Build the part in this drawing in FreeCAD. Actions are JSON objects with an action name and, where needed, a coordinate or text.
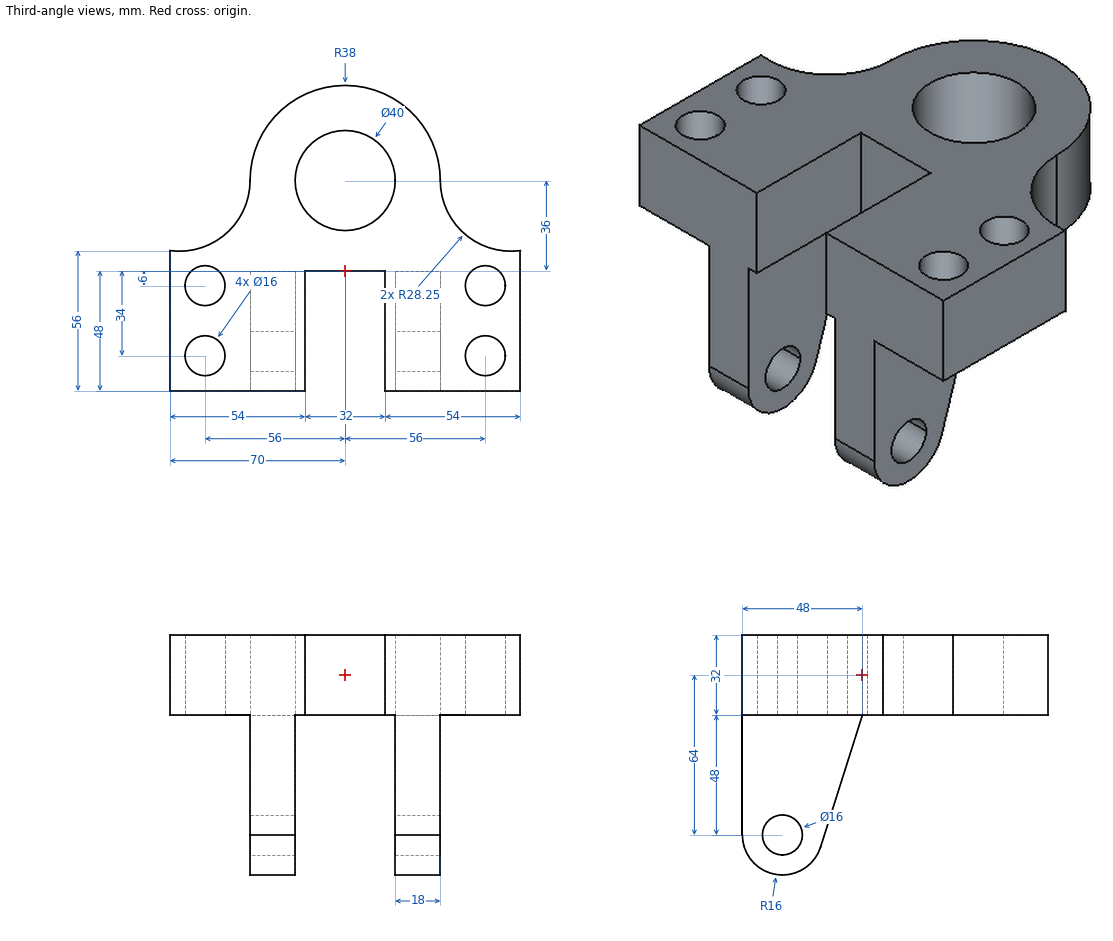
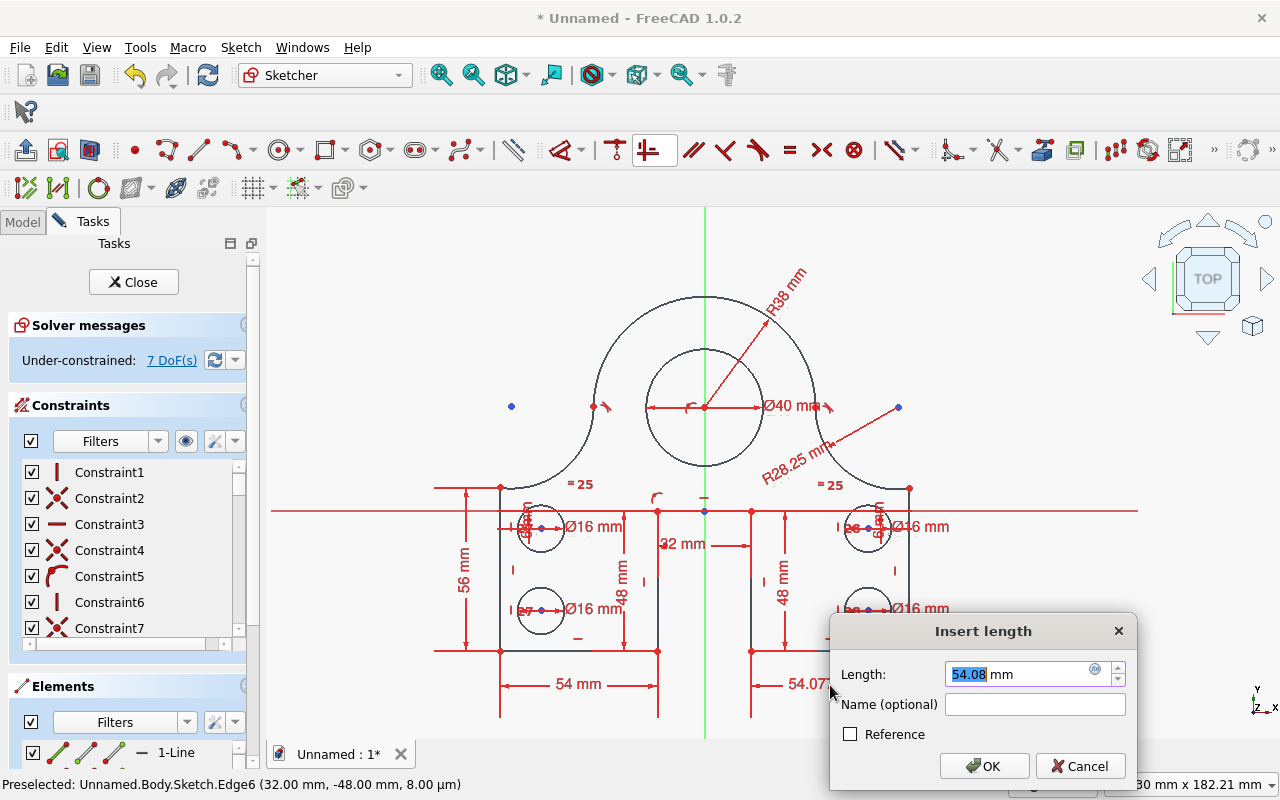
{"action": "type", "text": "54"}
{"action": "key", "text": "Return"}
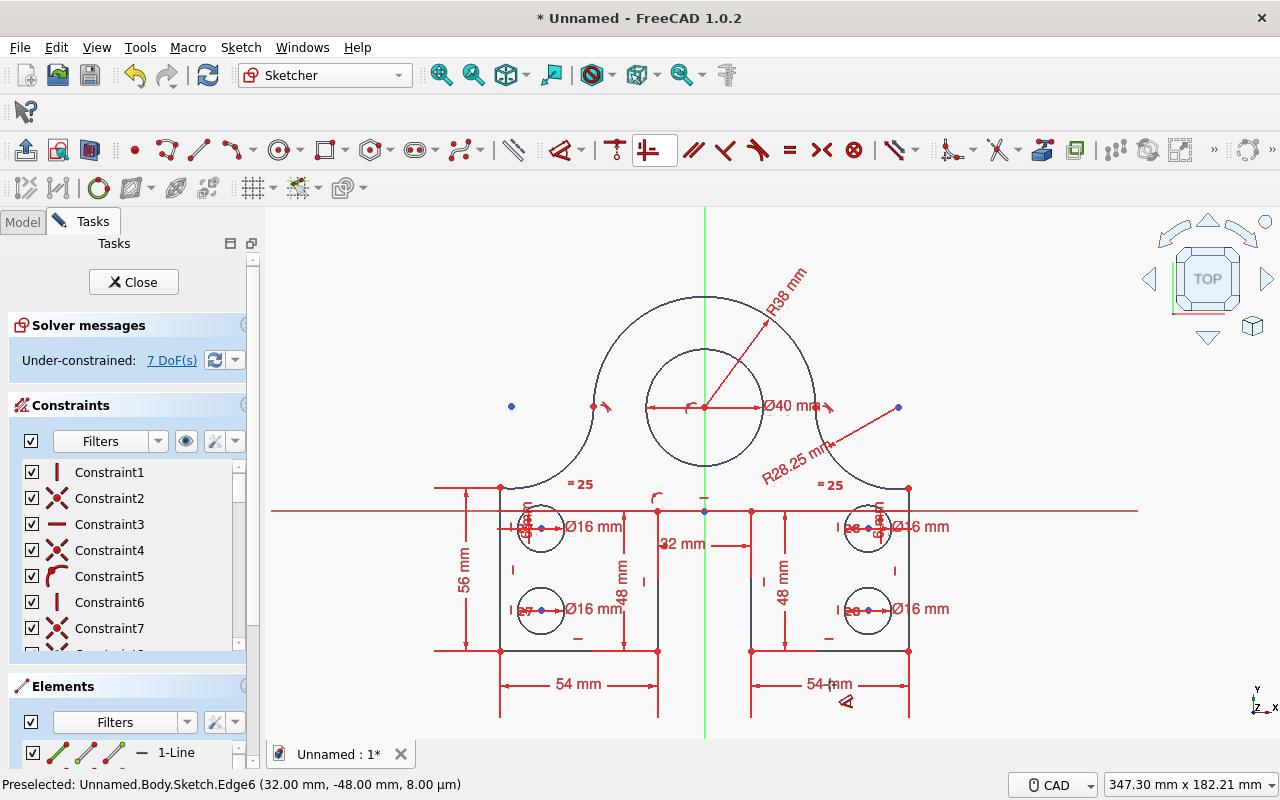
{"action": "left_click", "coordinate": [909, 603]}
{"action": "left_click", "coordinate": [943, 570]}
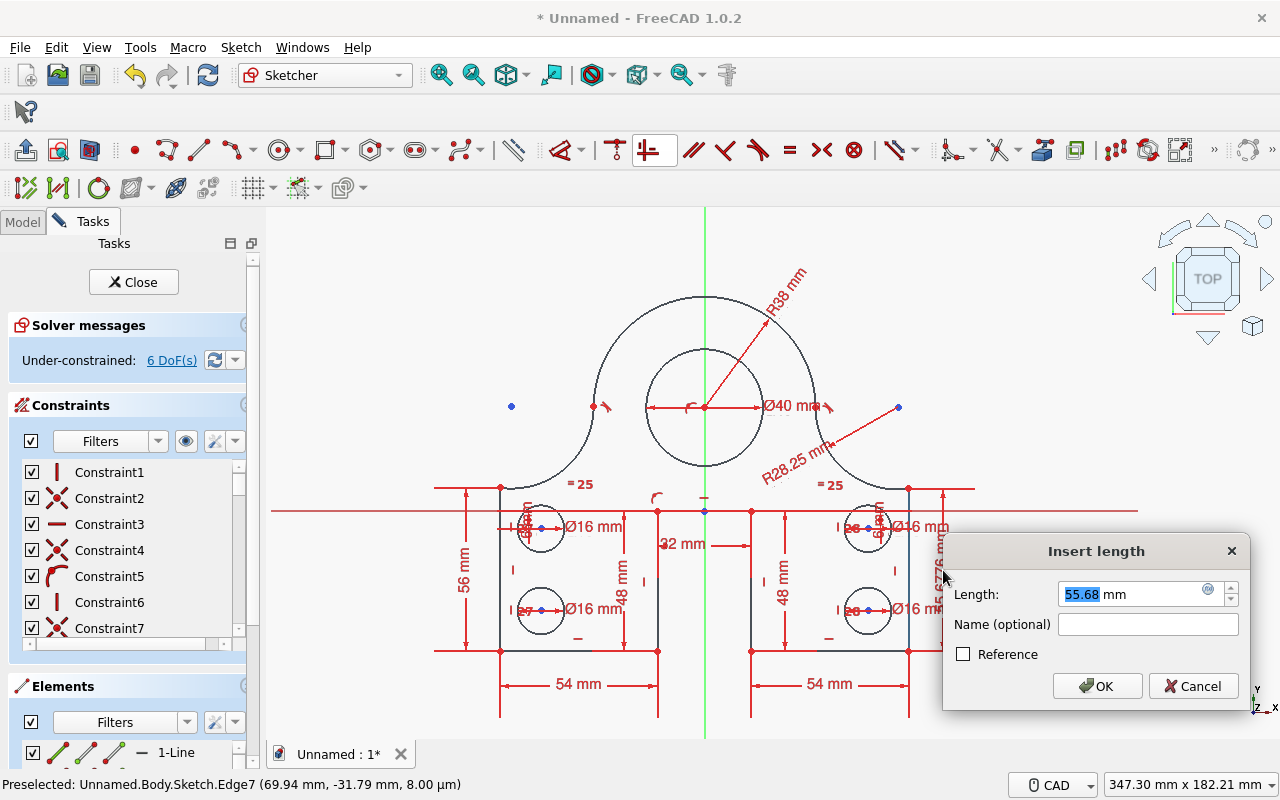
{"action": "type", "text": "56"}
{"action": "key", "text": "Return"}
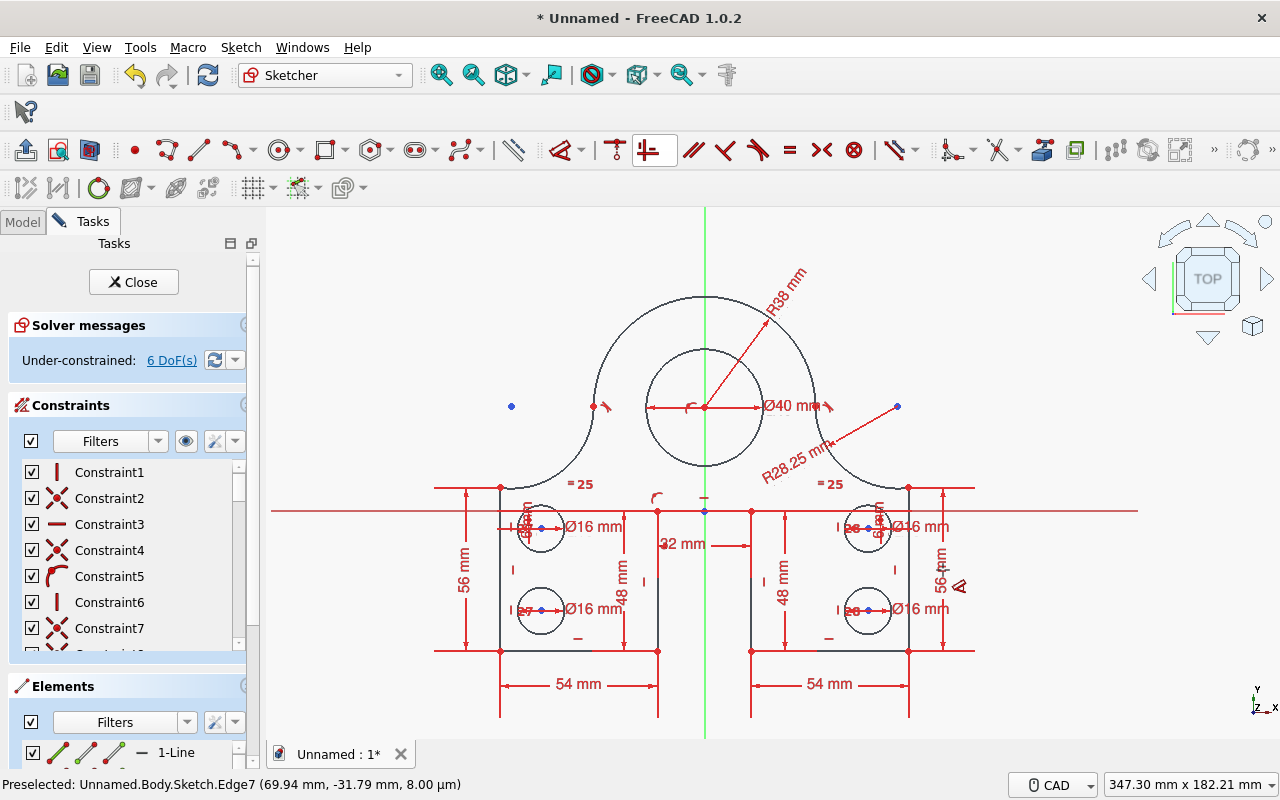
{"action": "left_click", "coordinate": [541, 611]}
{"action": "left_click", "coordinate": [680, 645]}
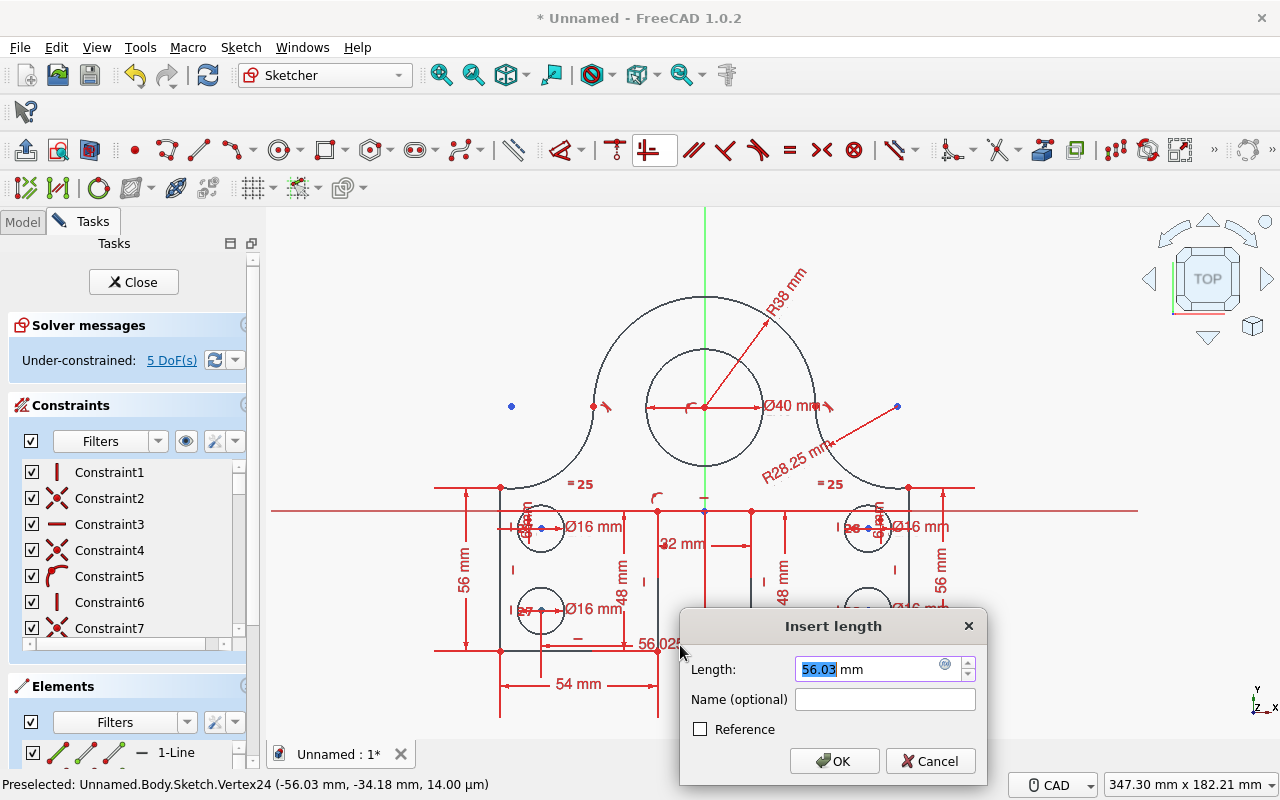
{"action": "type", "text": "56"}
{"action": "key", "text": "Return"}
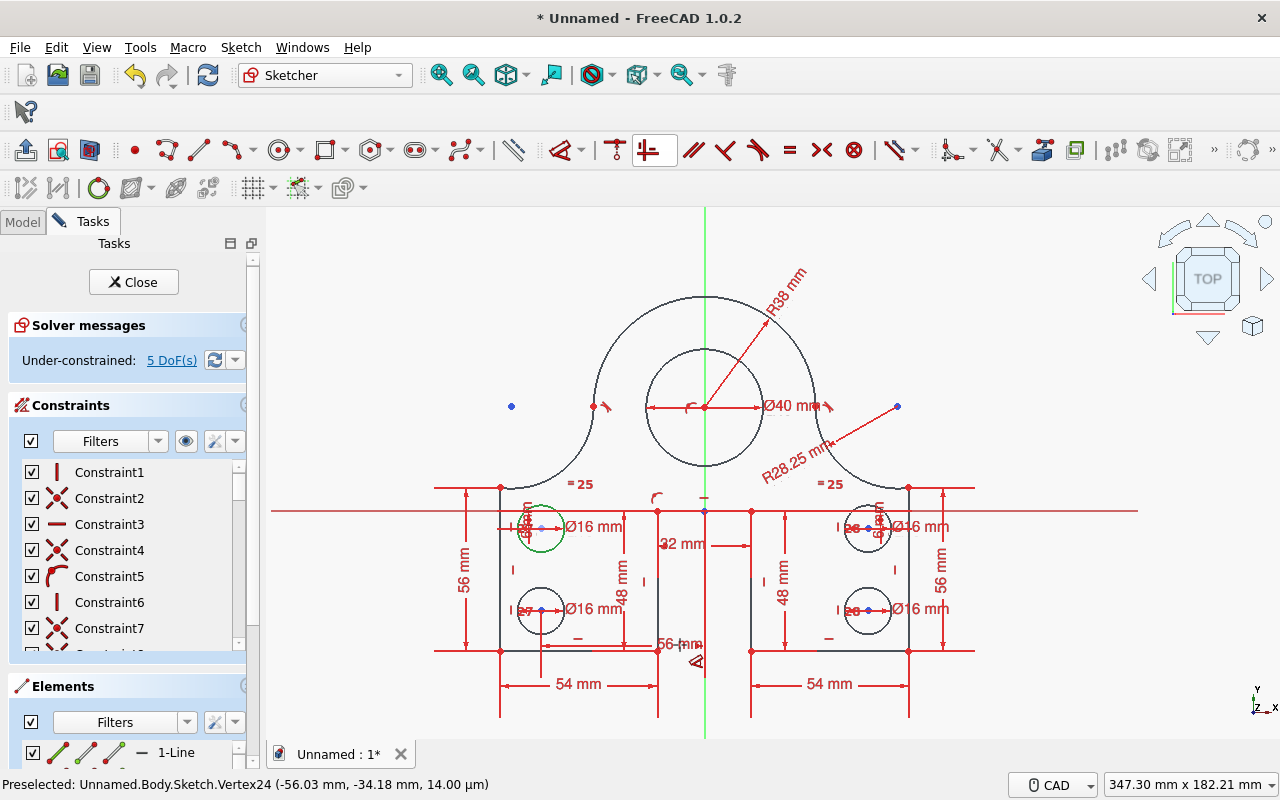
{"action": "left_click", "coordinate": [541, 611]}
{"action": "left_click", "coordinate": [483, 596]}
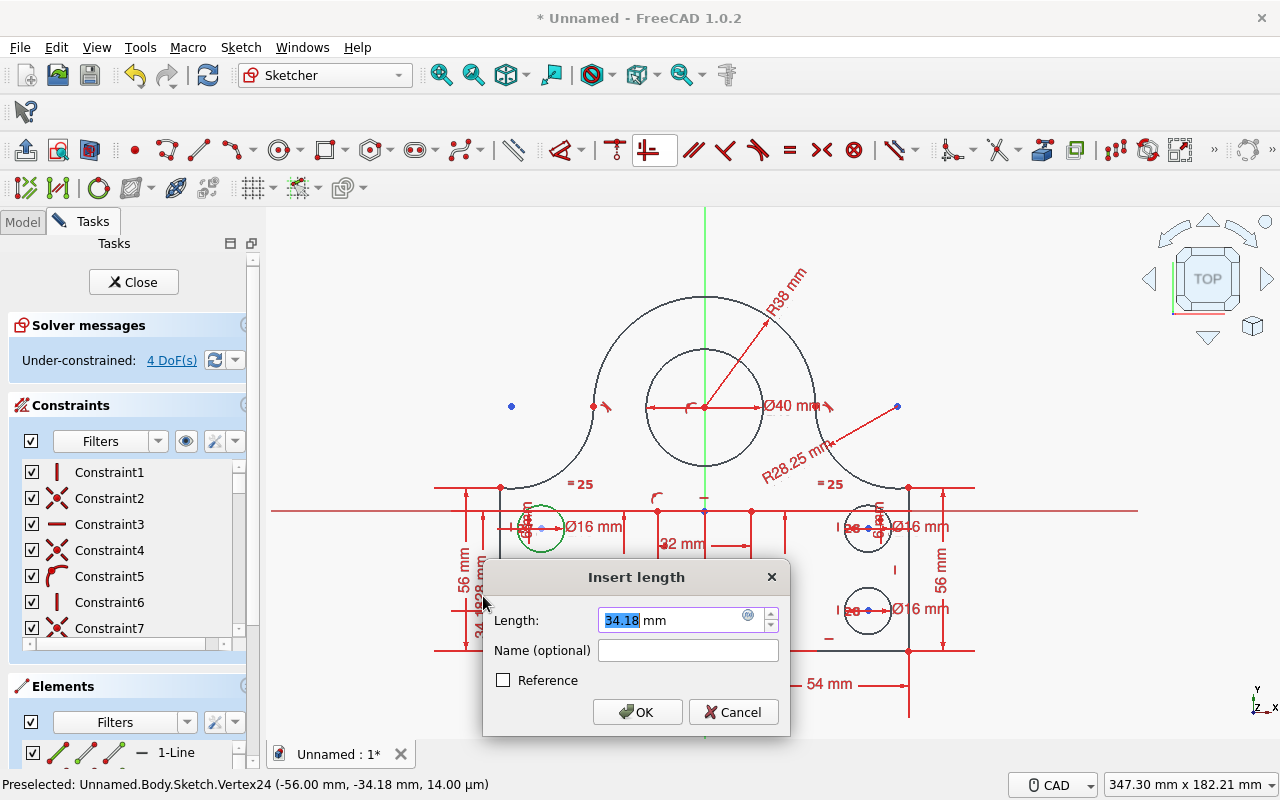
{"action": "type", "text": "34"}
{"action": "key", "text": "Return"}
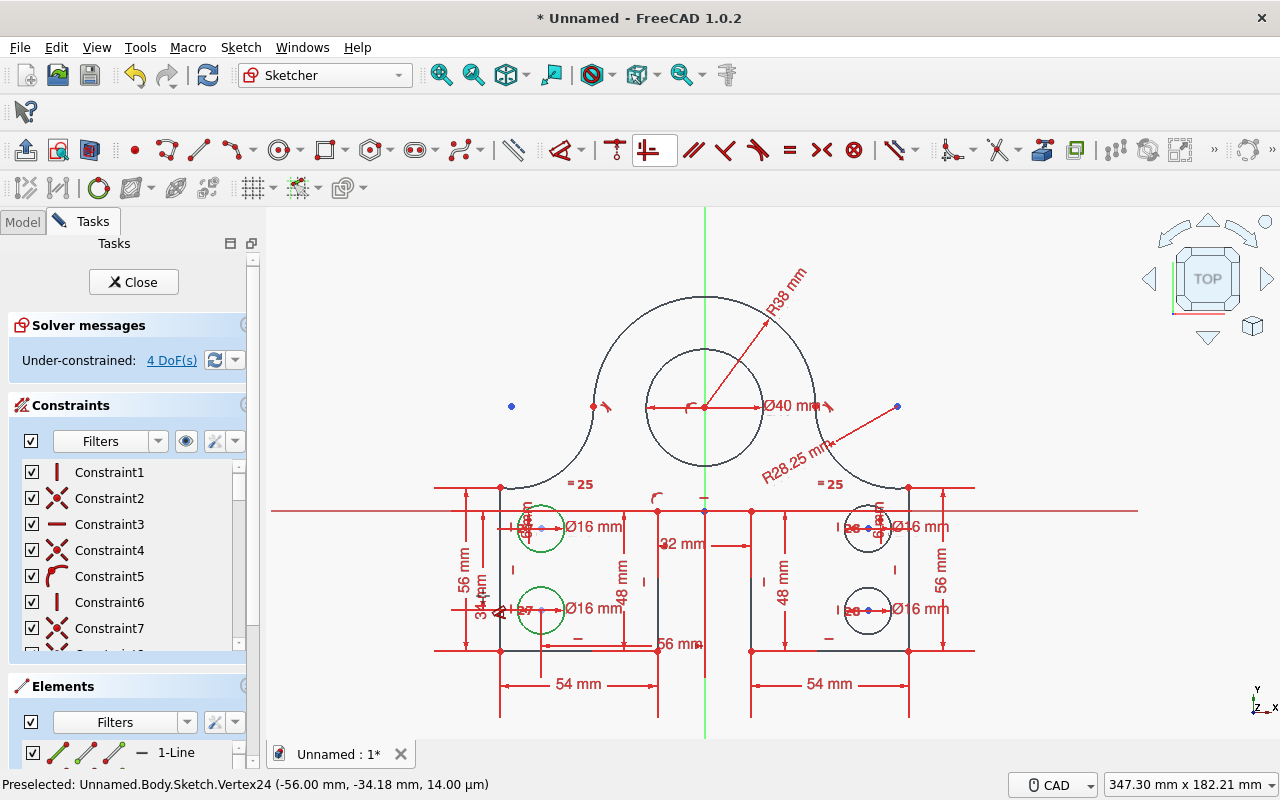
{"action": "left_click", "coordinate": [868, 611]}
{"action": "left_click", "coordinate": [749, 669]}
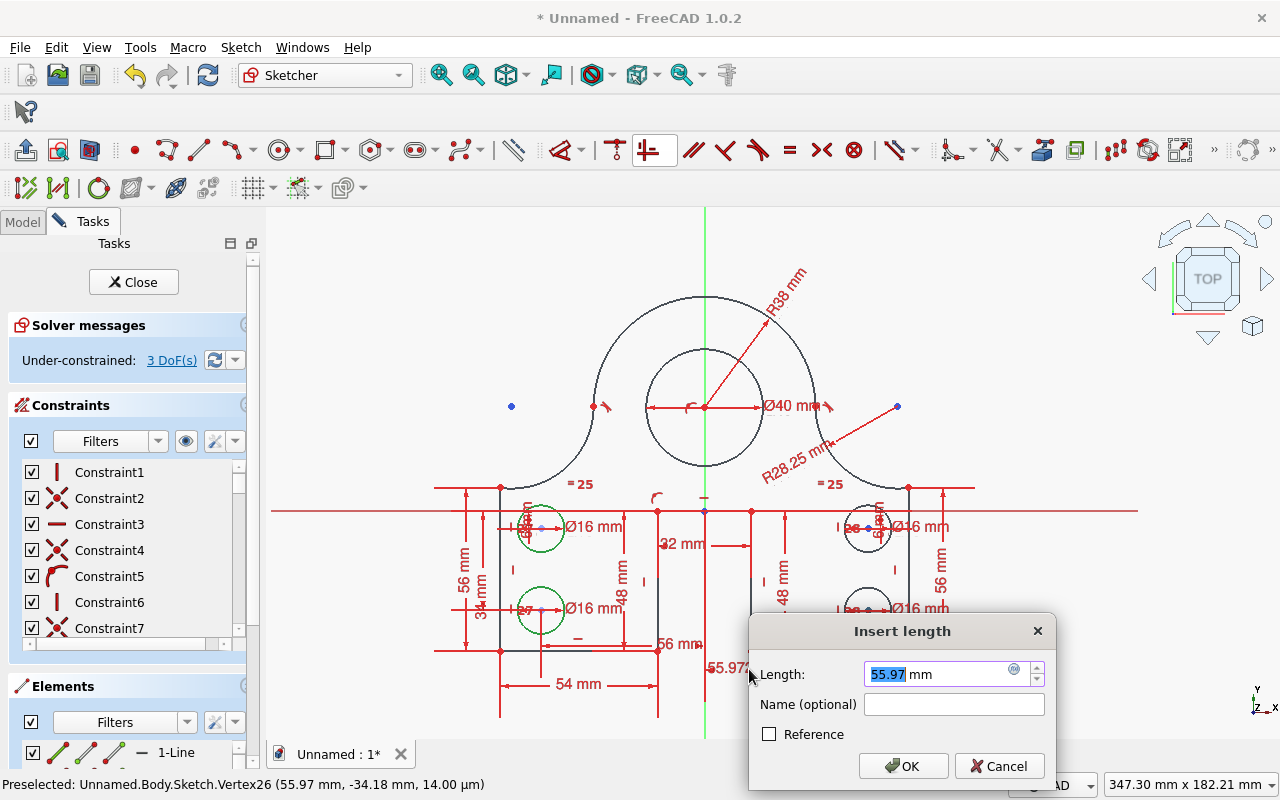
{"action": "type", "text": "56"}
{"action": "key", "text": "Return"}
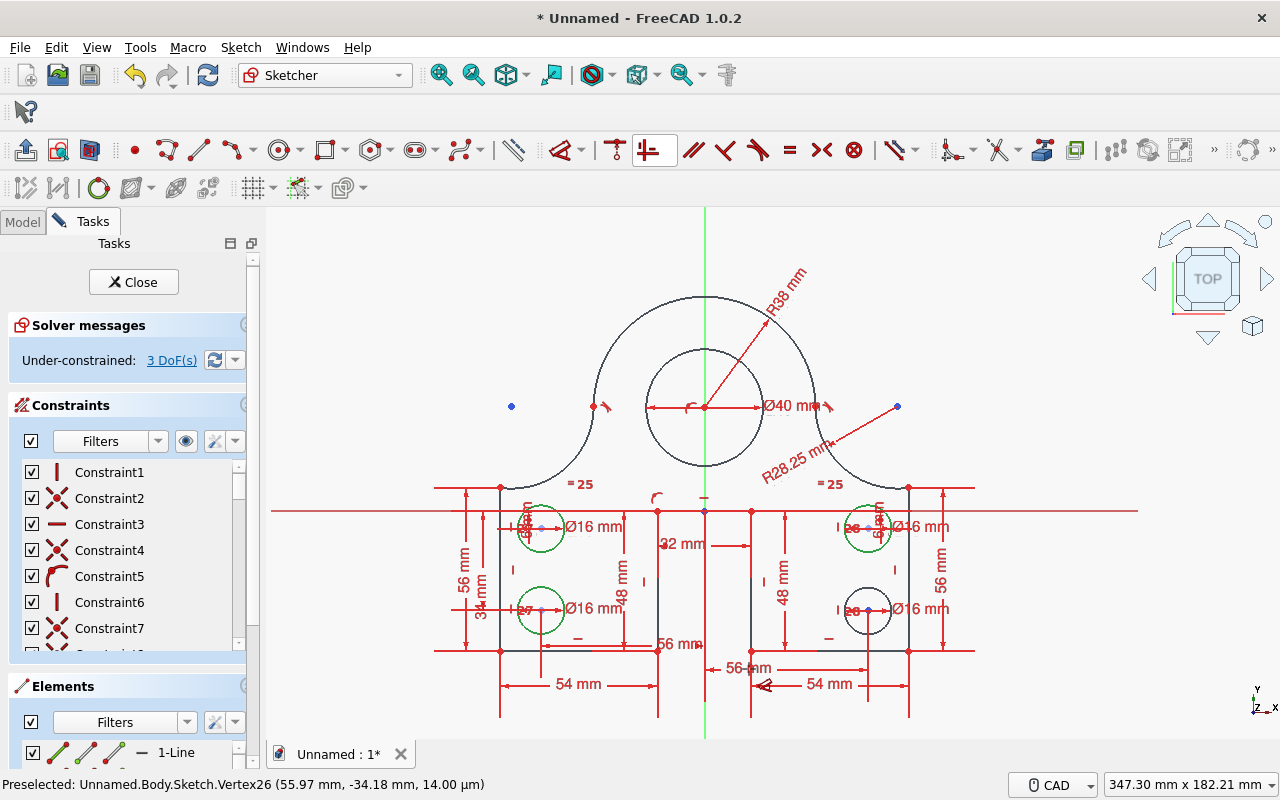
{"action": "left_click", "coordinate": [868, 611]}
{"action": "left_click", "coordinate": [926, 596]}